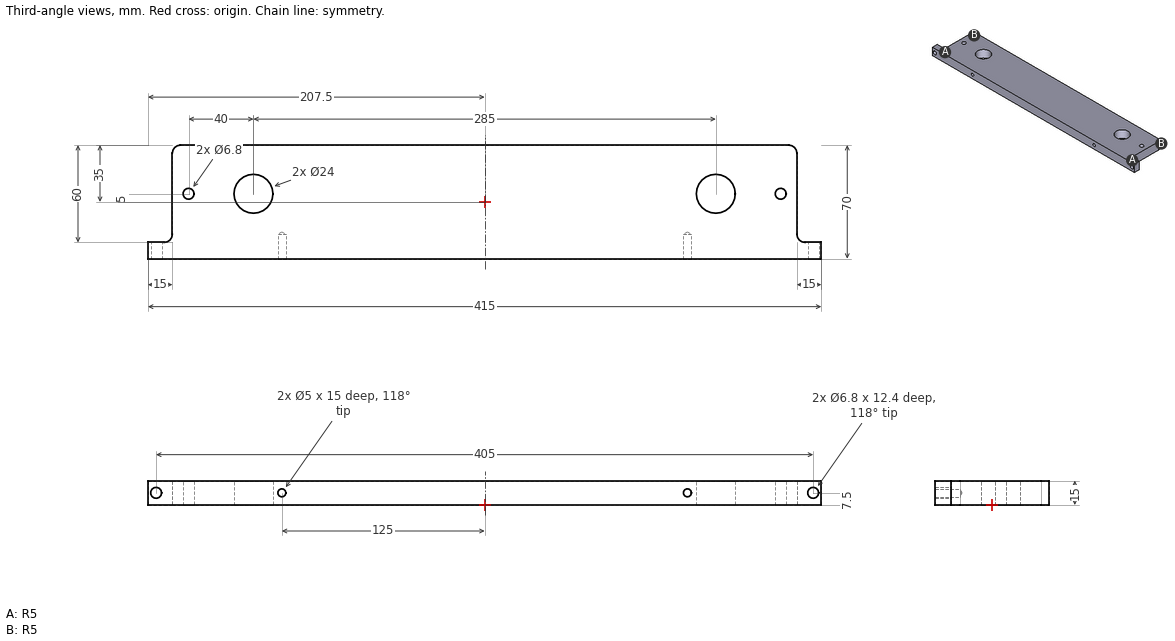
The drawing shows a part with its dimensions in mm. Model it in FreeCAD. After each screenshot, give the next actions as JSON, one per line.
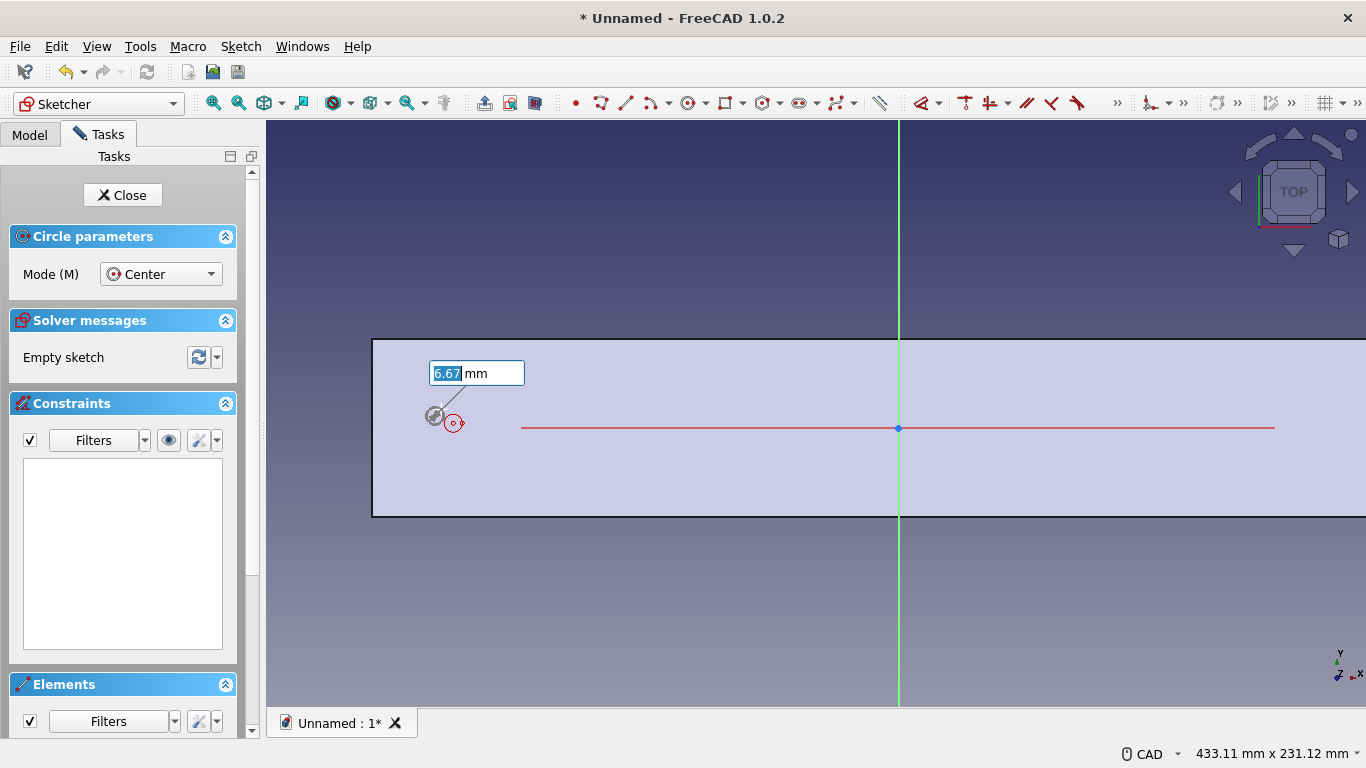
{"action": "type", "text": "6.8"}
{"action": "key", "text": "Return"}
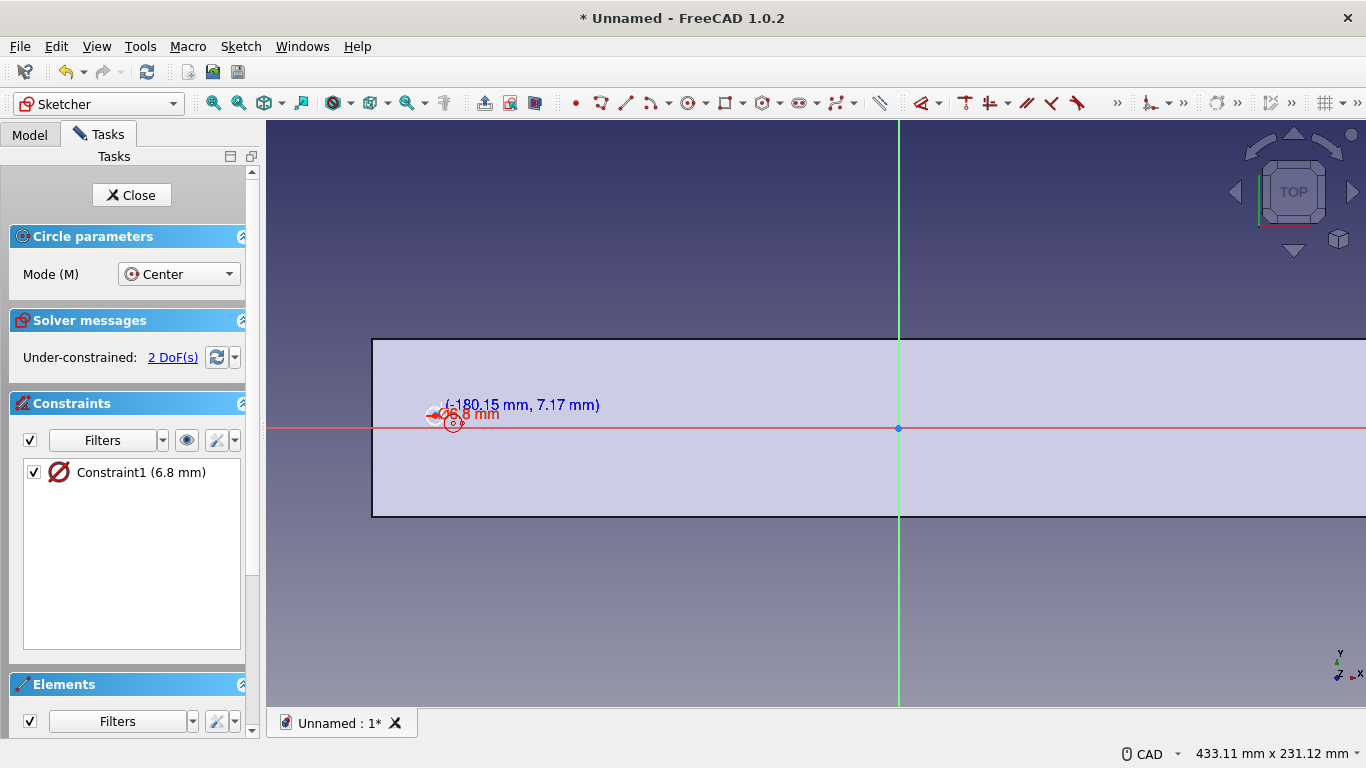
{"action": "scroll", "coordinate": [537, 416], "scroll_direction": "up", "scroll_amount": 2}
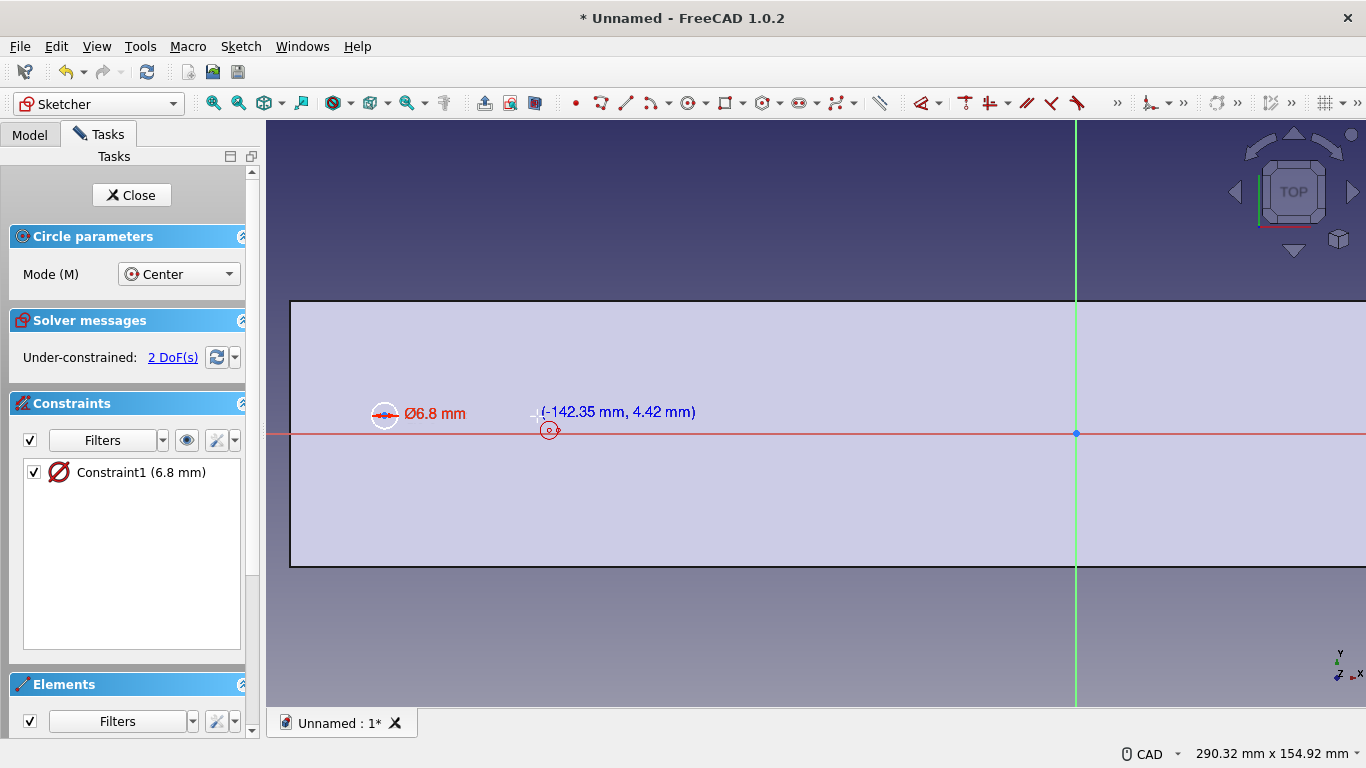
{"action": "left_click", "coordinate": [536, 415]}
{"action": "mouse_move", "coordinate": [568, 383]}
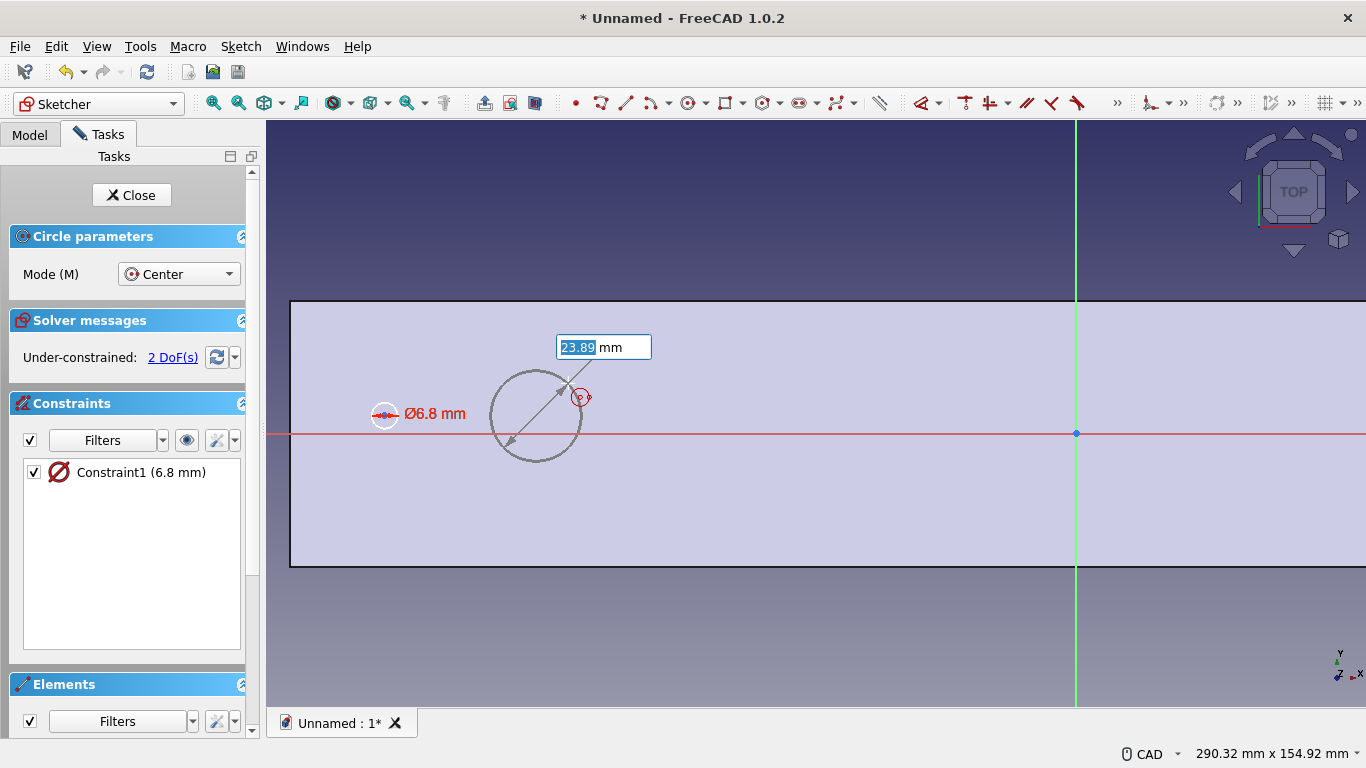
{"action": "type", "text": "24"}
{"action": "key", "text": "Return"}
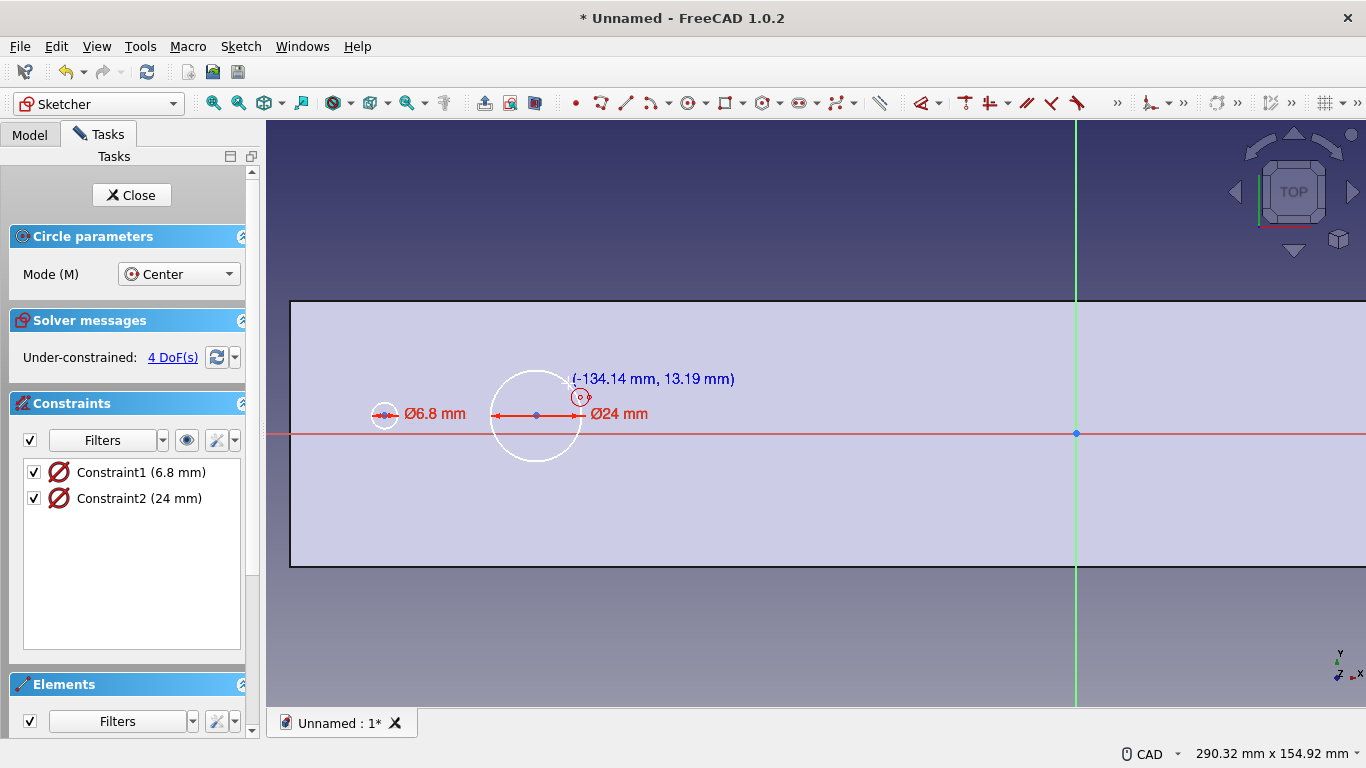
{"action": "scroll", "coordinate": [479, 412], "scroll_direction": "down", "scroll_amount": 4}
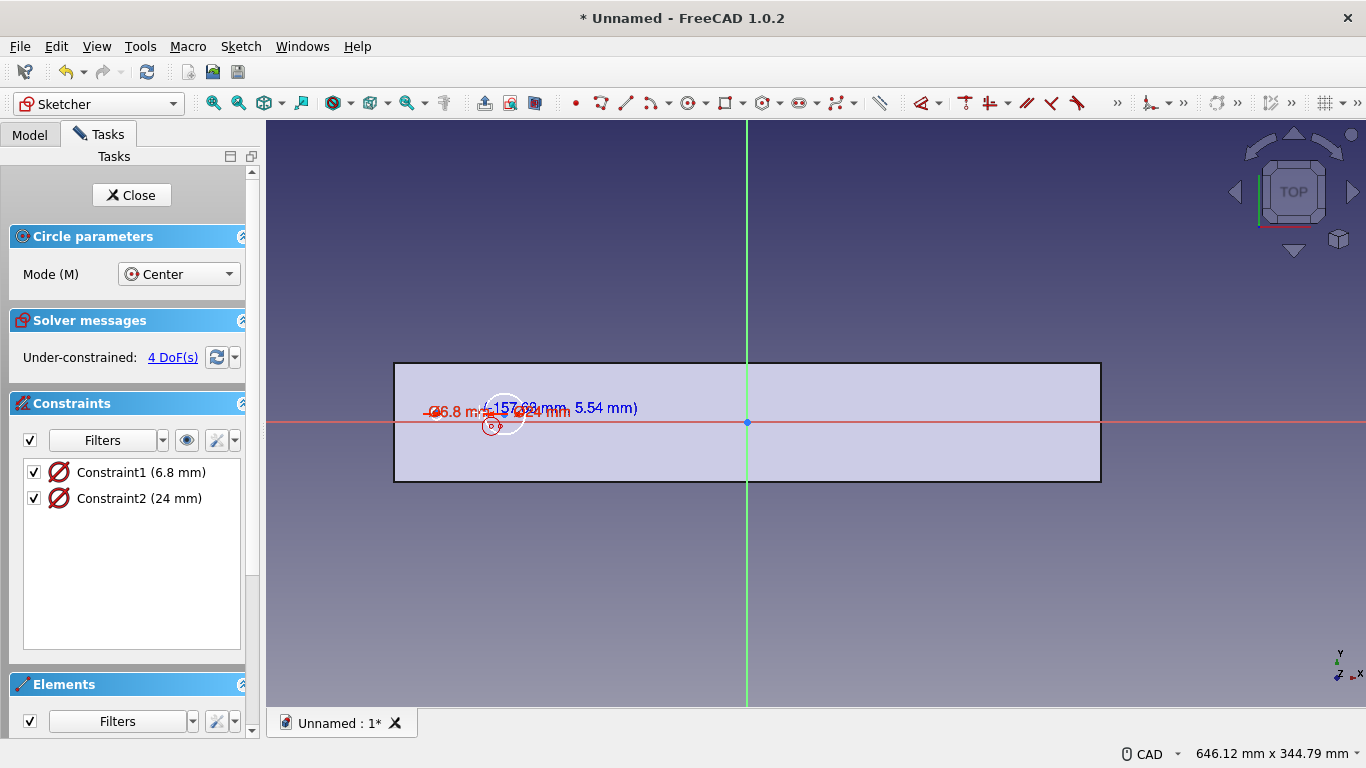
{"action": "scroll", "coordinate": [990, 414], "scroll_direction": "up", "scroll_amount": 4}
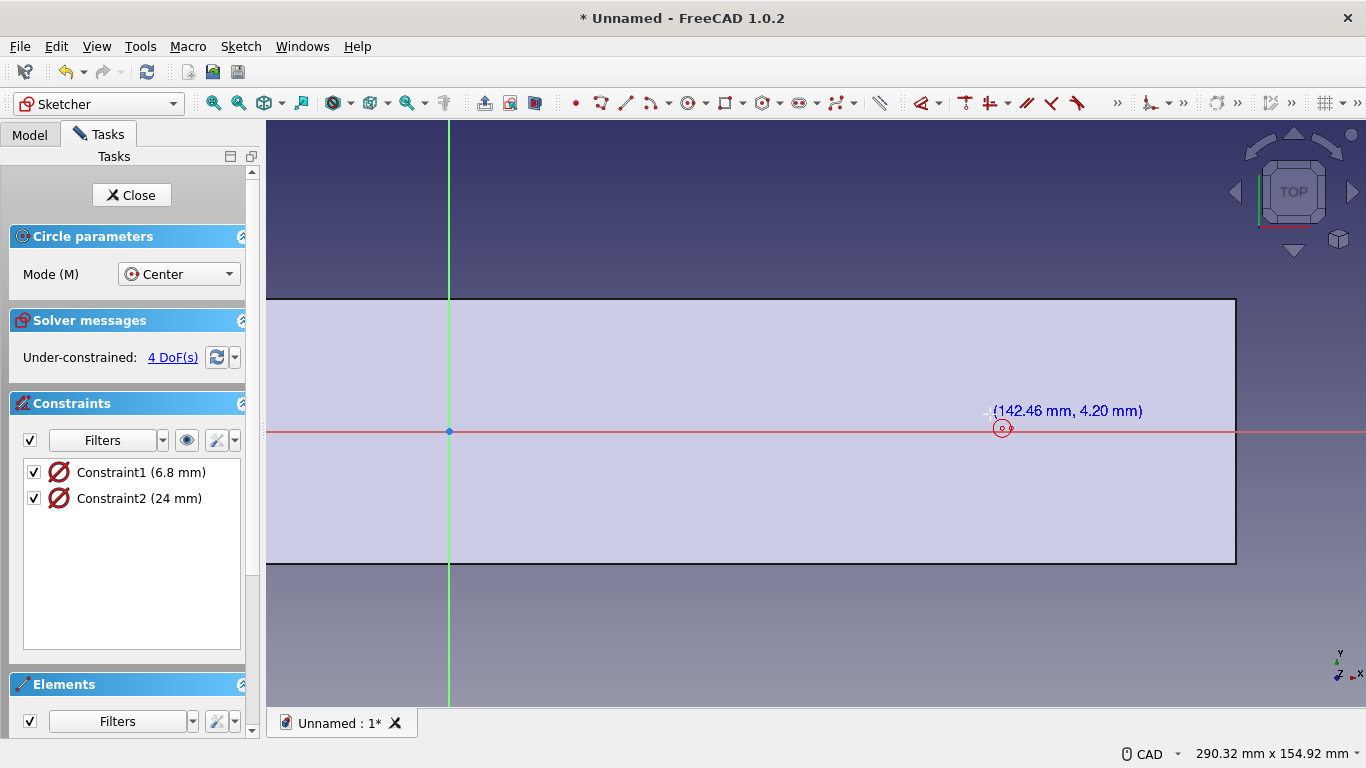
{"action": "left_click", "coordinate": [989, 413]}
{"action": "mouse_move", "coordinate": [1021, 380]}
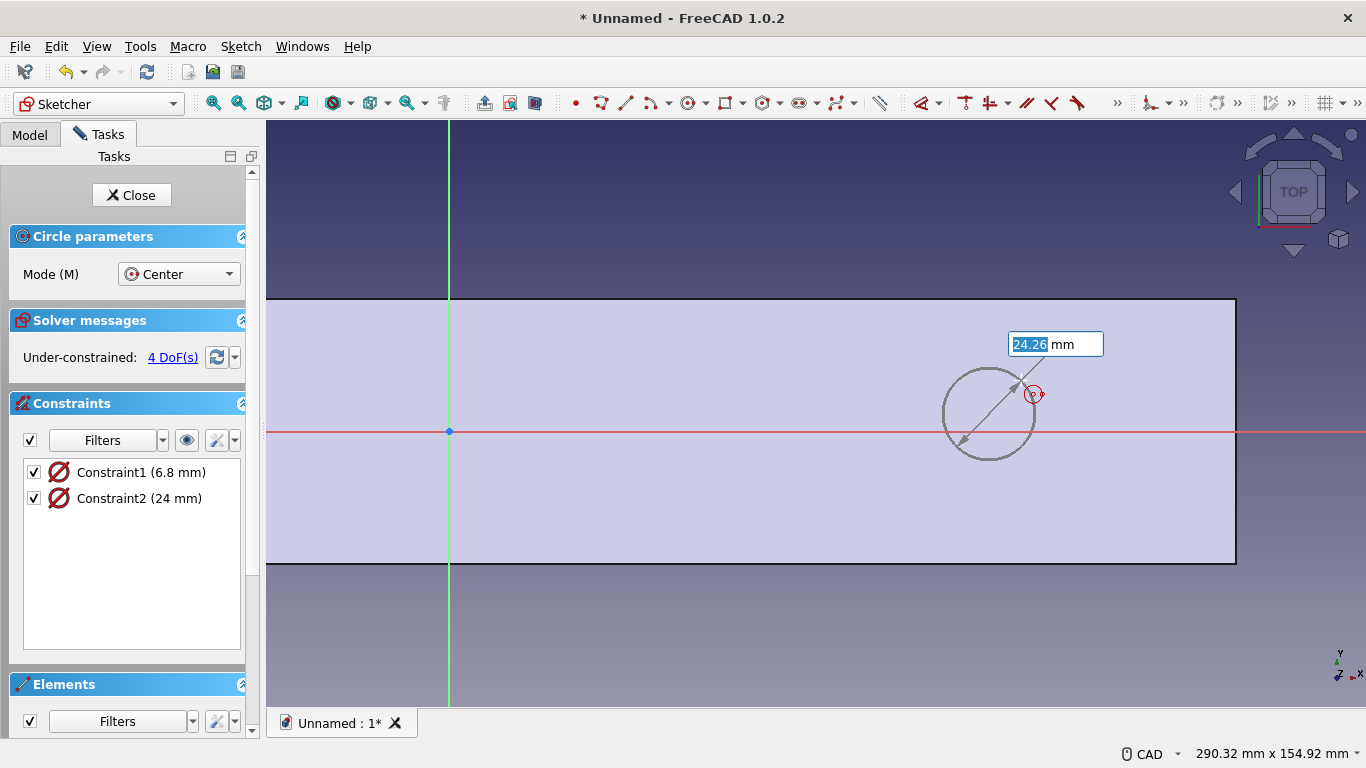
{"action": "type", "text": "24"}
{"action": "key", "text": "Return"}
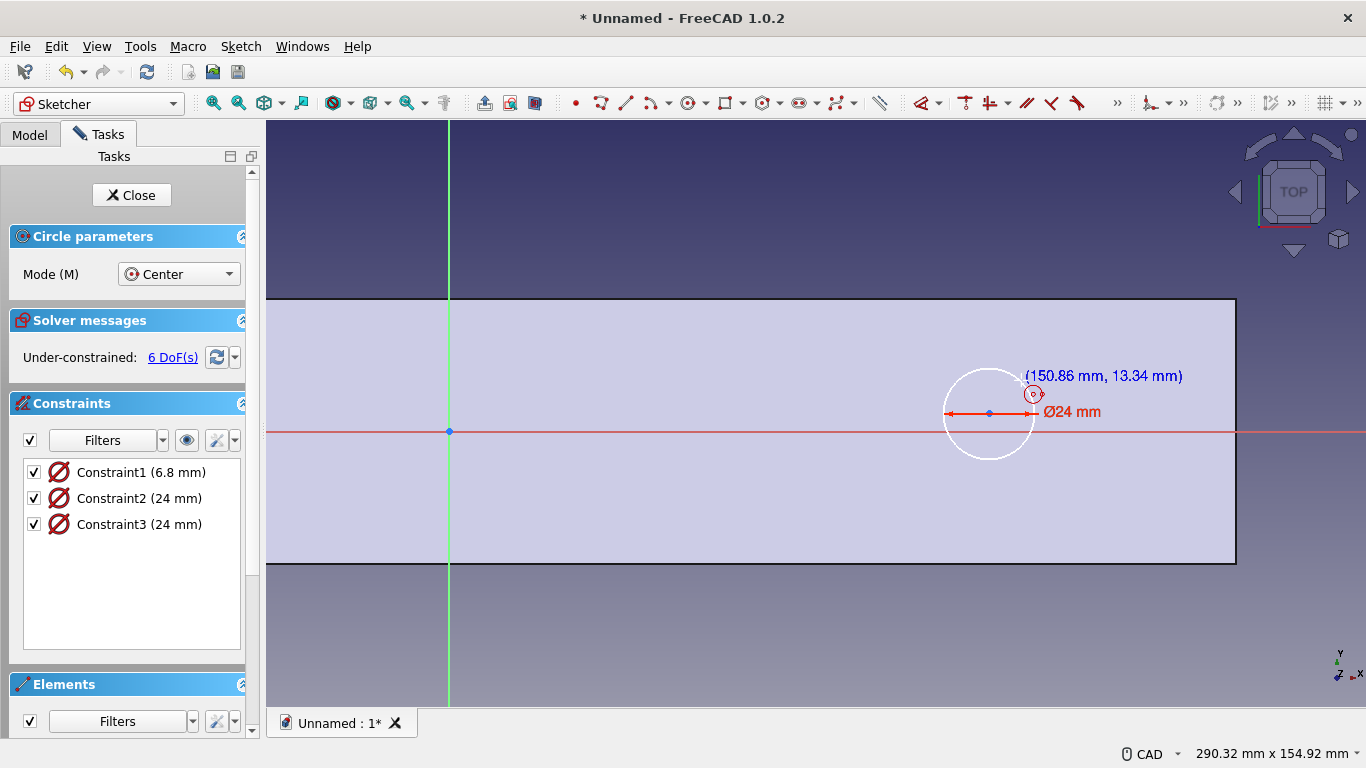
{"action": "scroll", "coordinate": [1141, 413], "scroll_direction": "up", "scroll_amount": 3}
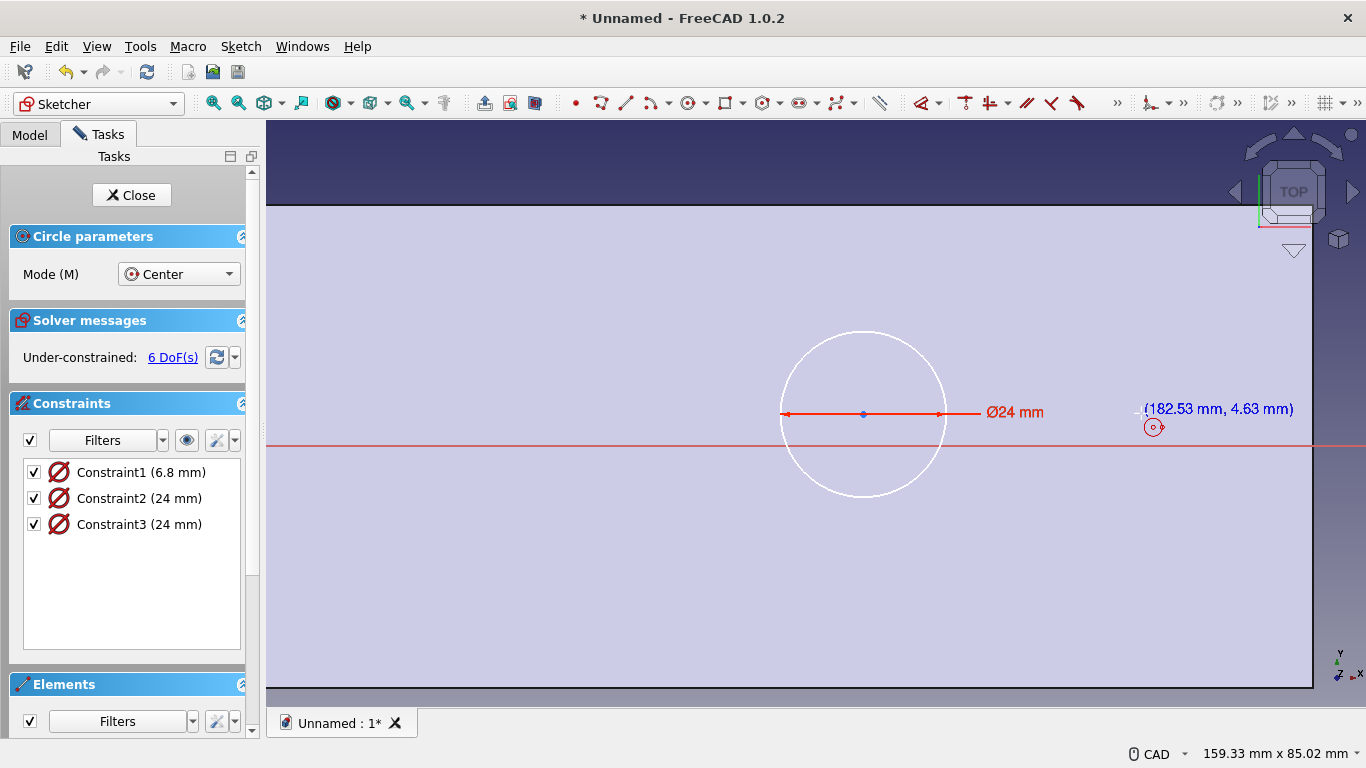
{"action": "left_click", "coordinate": [1140, 412]}